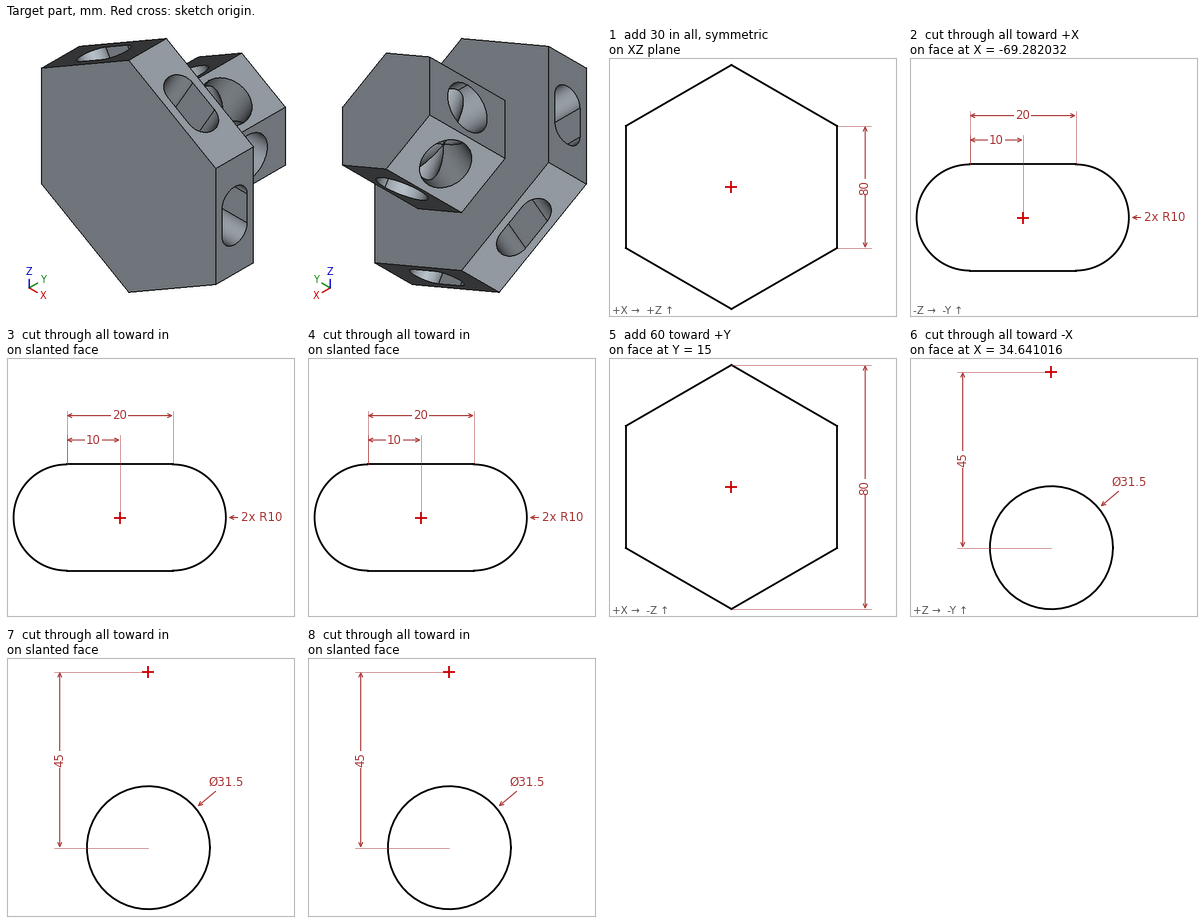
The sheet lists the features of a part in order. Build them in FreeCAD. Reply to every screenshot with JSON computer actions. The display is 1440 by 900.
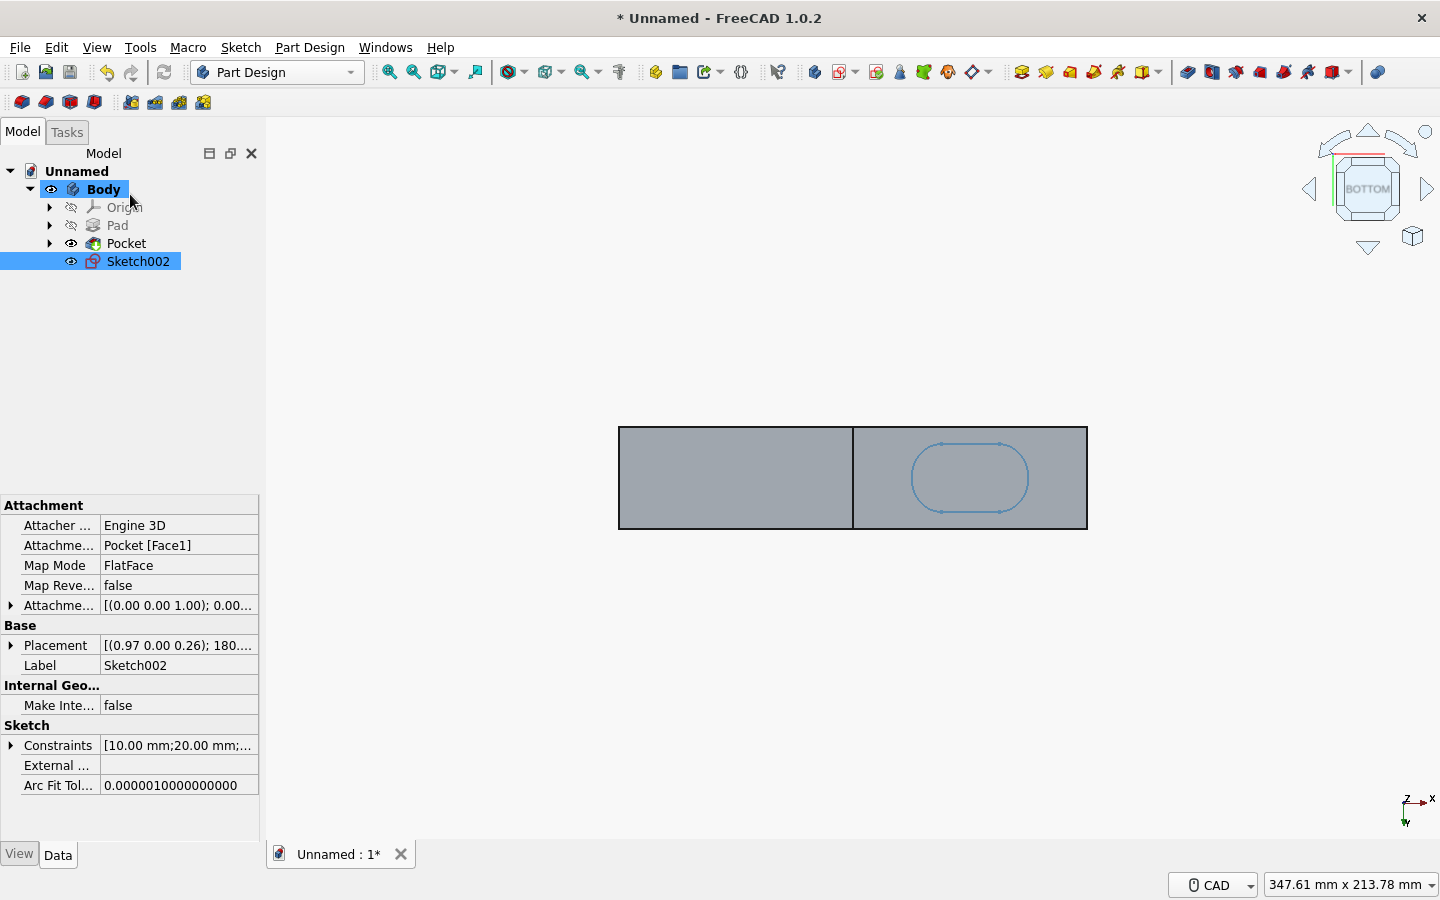
{"action": "left_click", "coordinate": [1188, 72]}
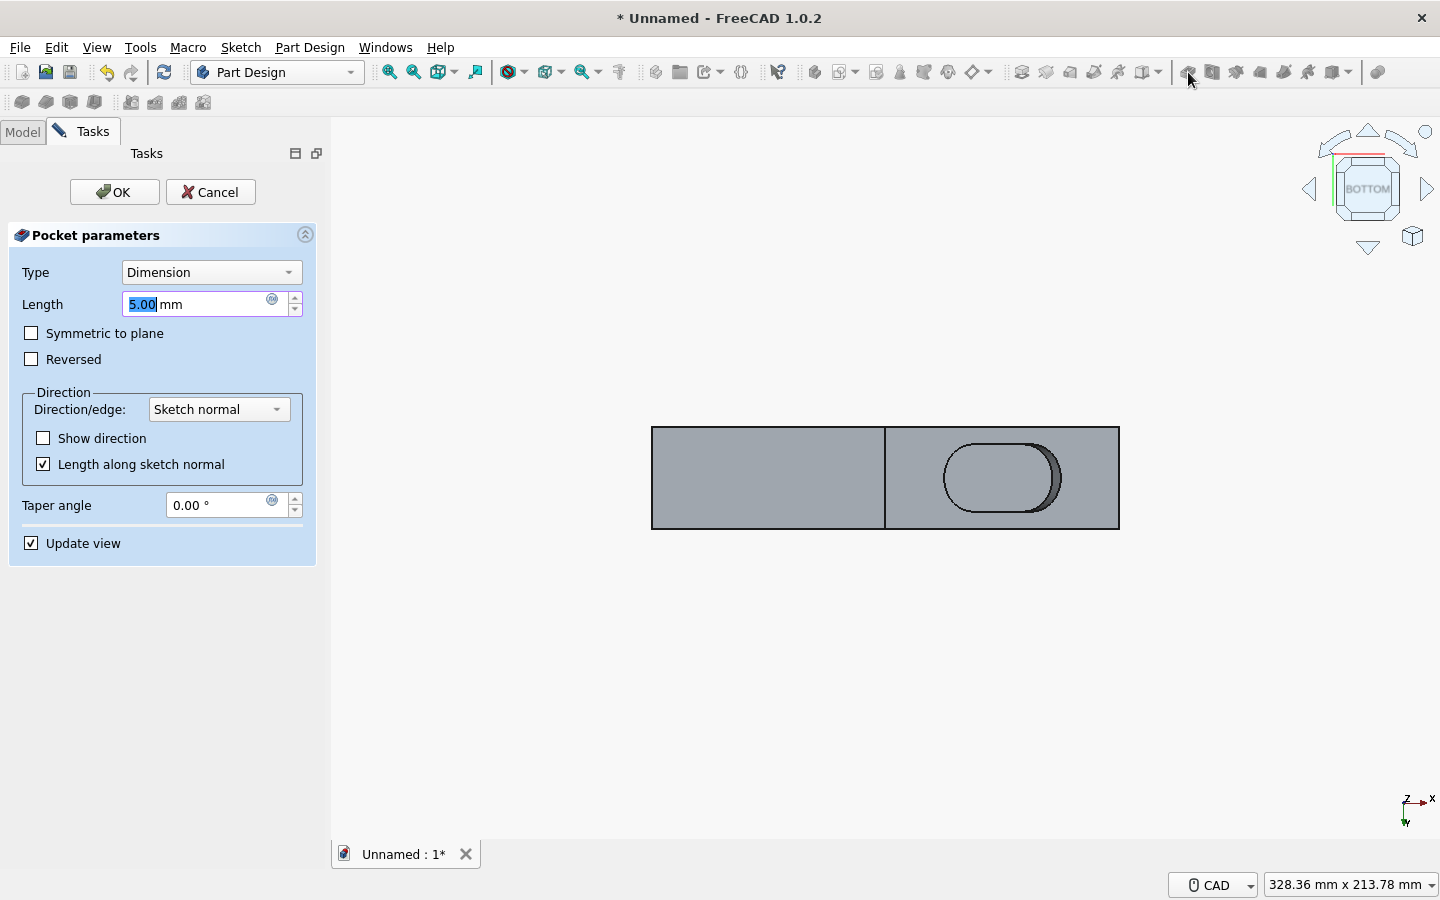
{"action": "left_click", "coordinate": [212, 272]}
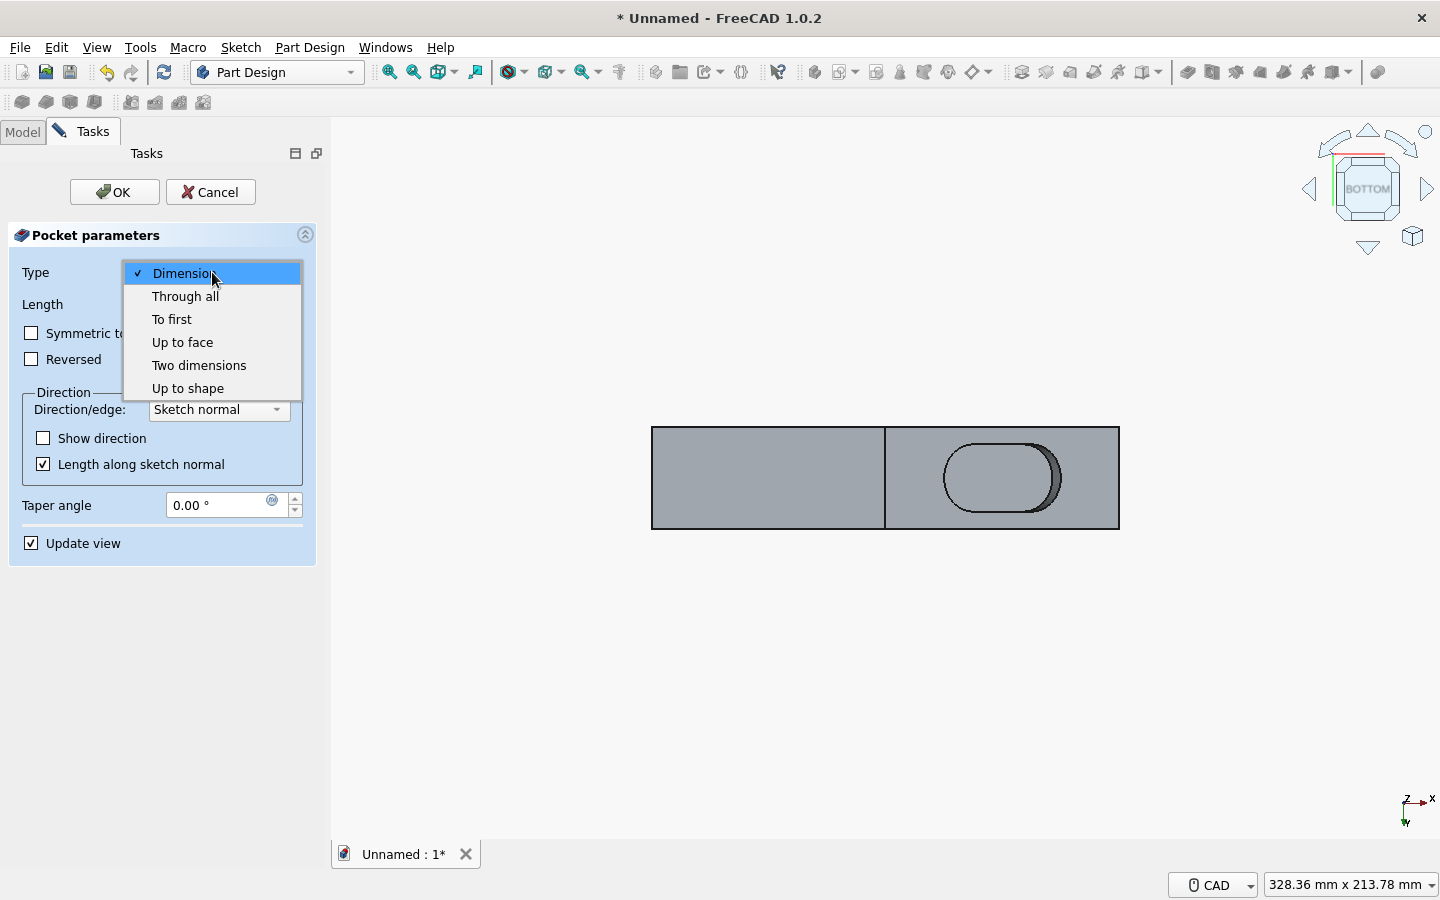
{"action": "left_click", "coordinate": [212, 296]}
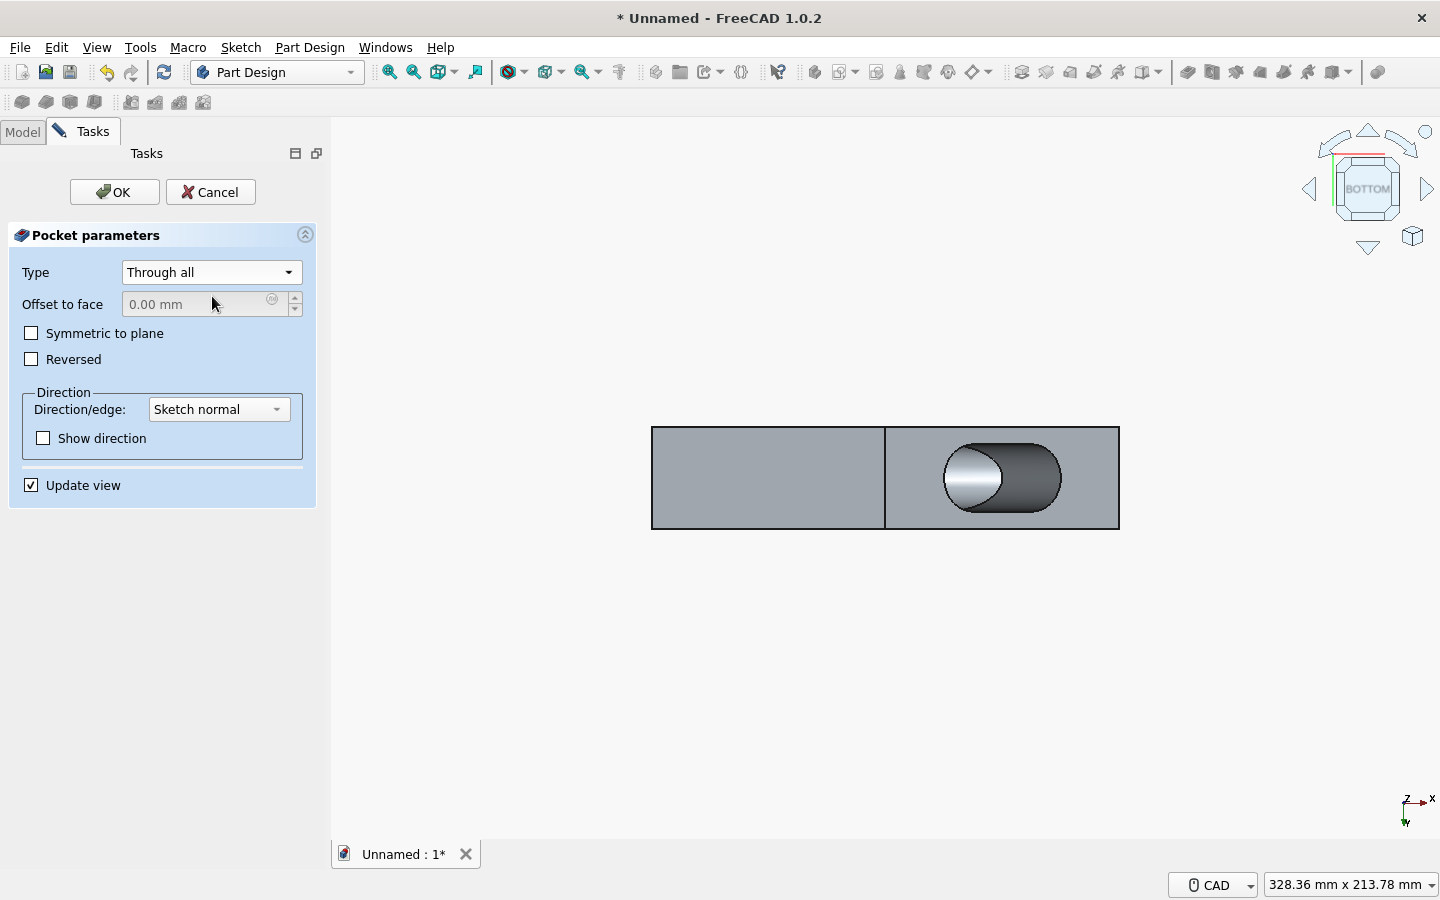
{"action": "left_click", "coordinate": [115, 192]}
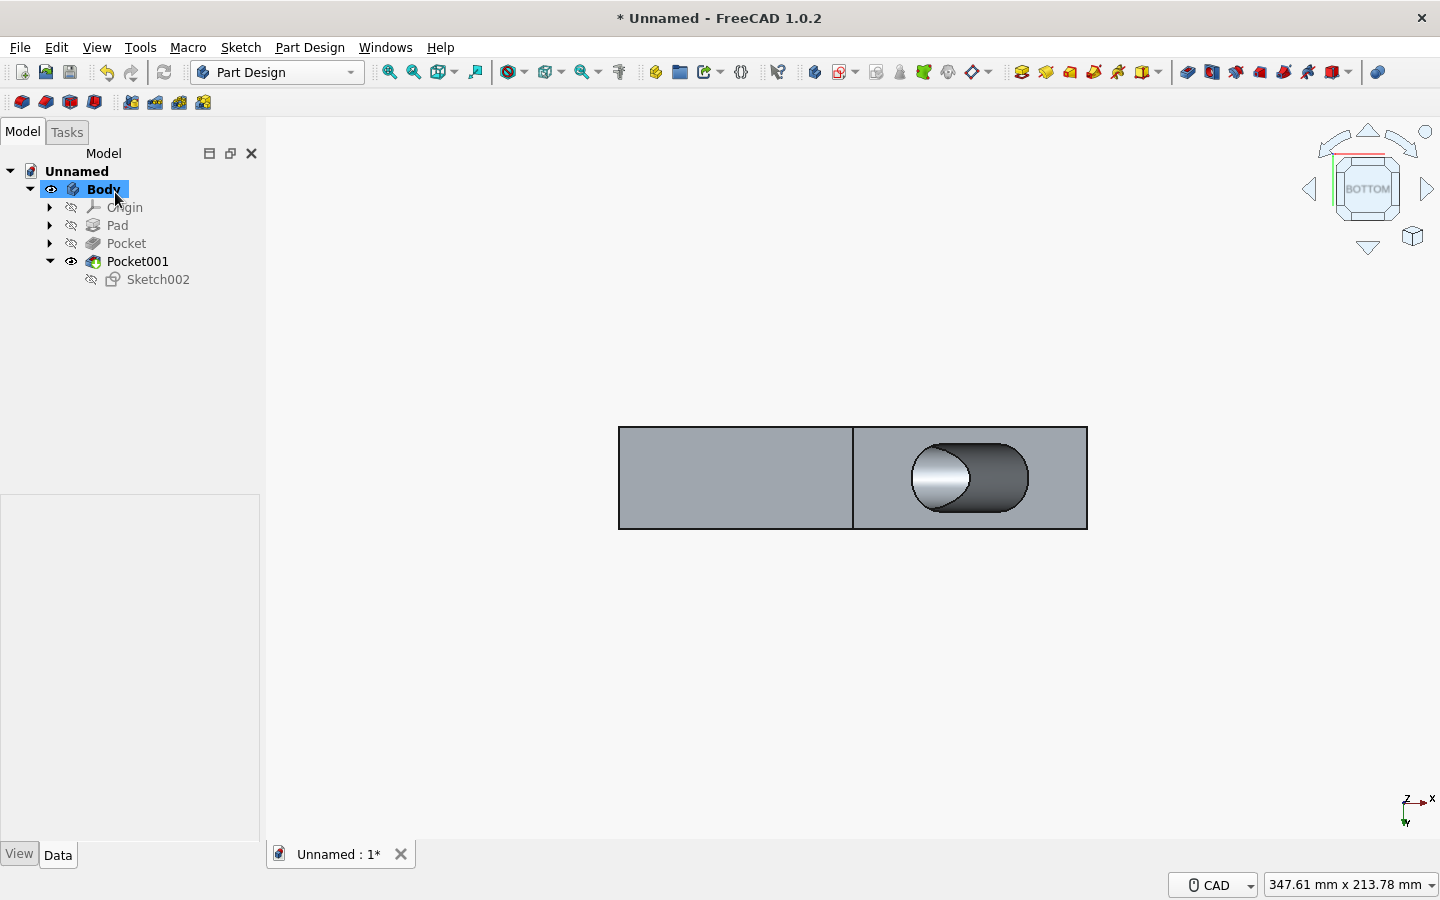
{"action": "left_click", "coordinate": [390, 72]}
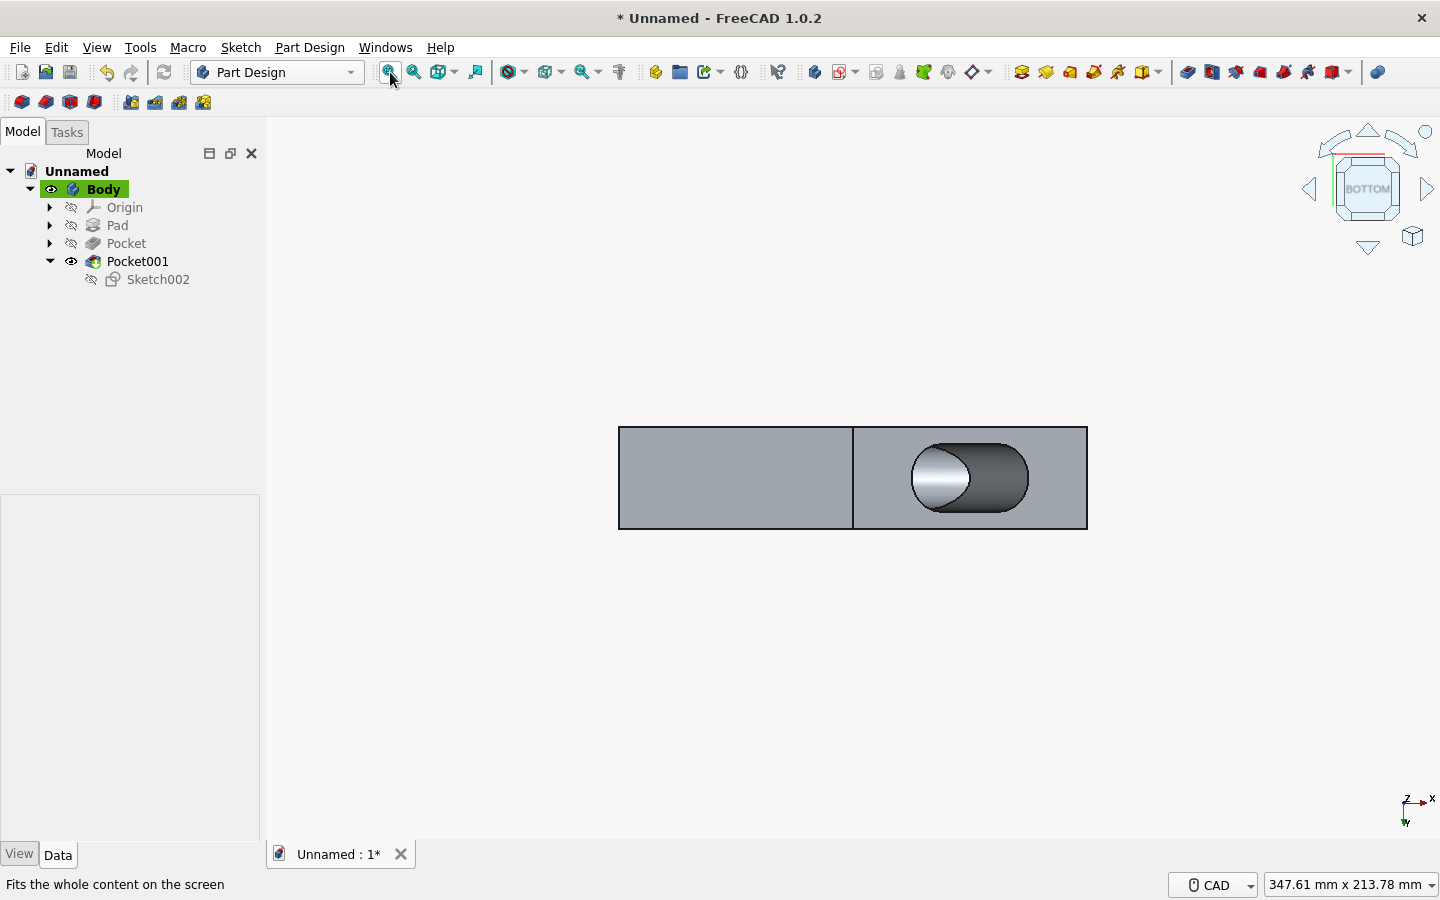
{"action": "left_click", "coordinate": [803, 477]}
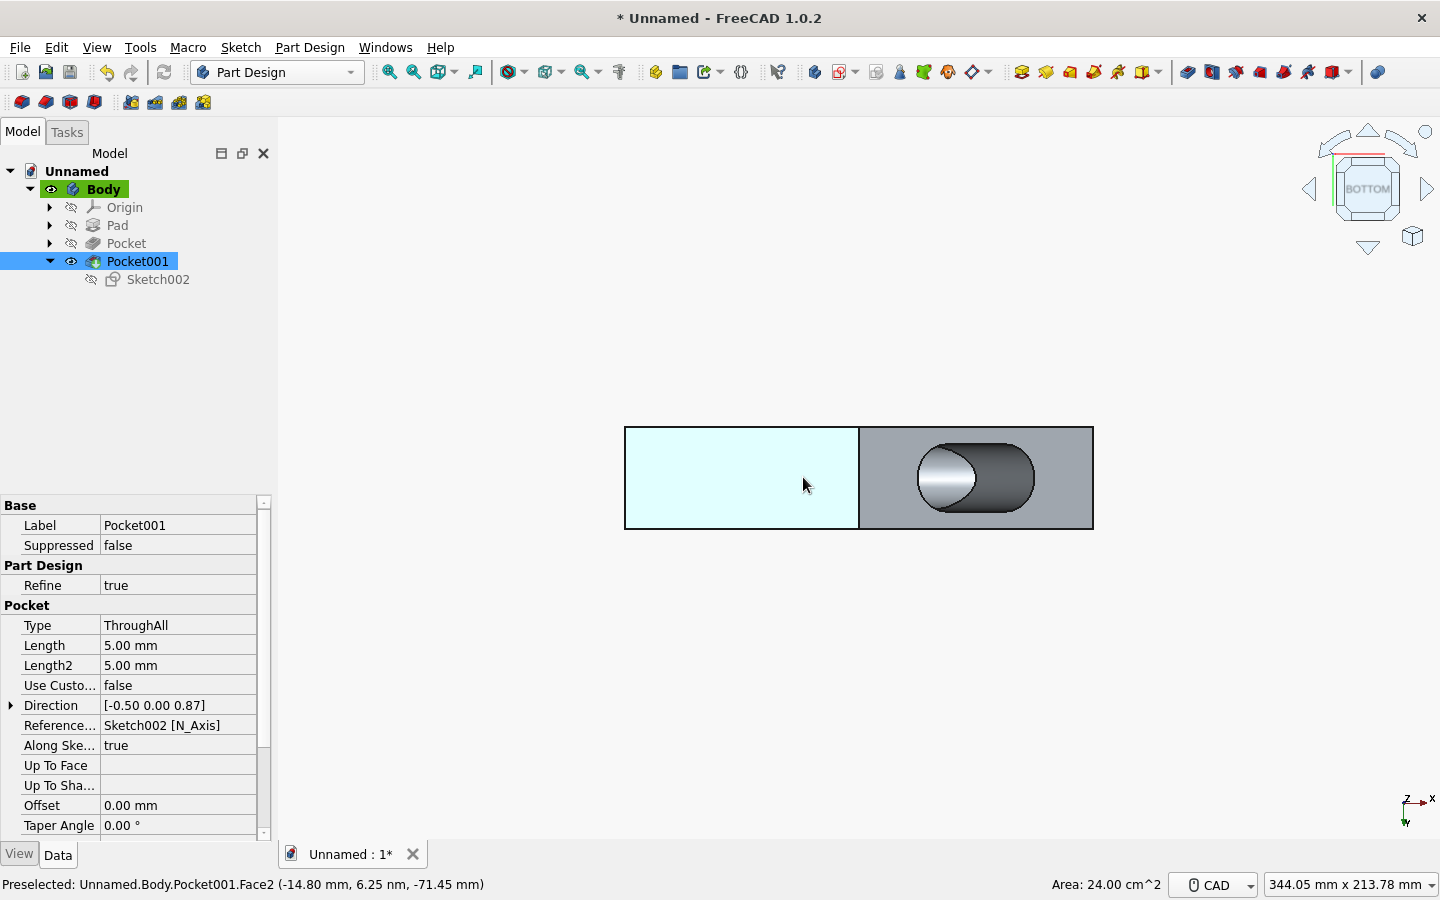
{"action": "left_click", "coordinate": [840, 72]}